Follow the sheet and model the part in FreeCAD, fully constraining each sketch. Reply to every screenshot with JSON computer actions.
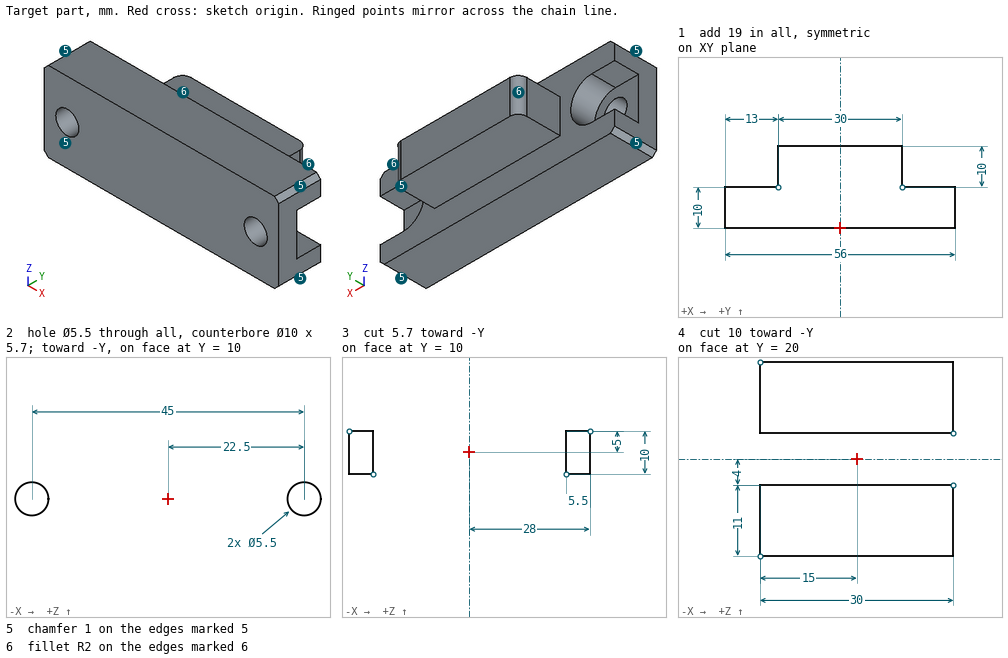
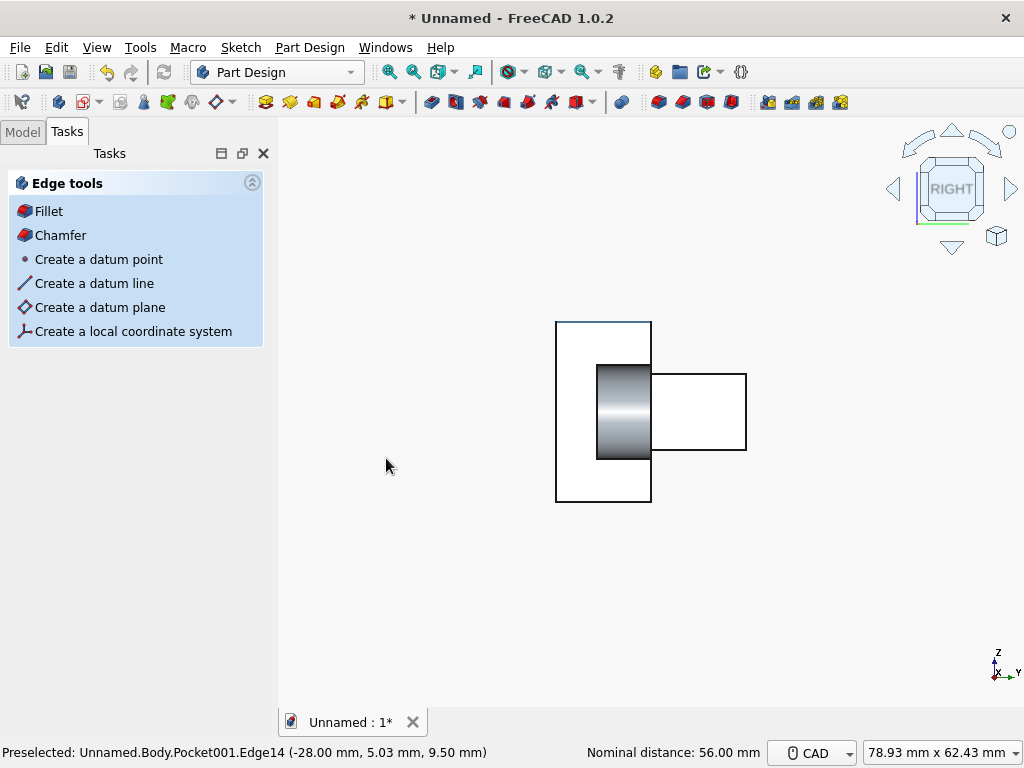
{"action": "left_click", "coordinate": [390, 72]}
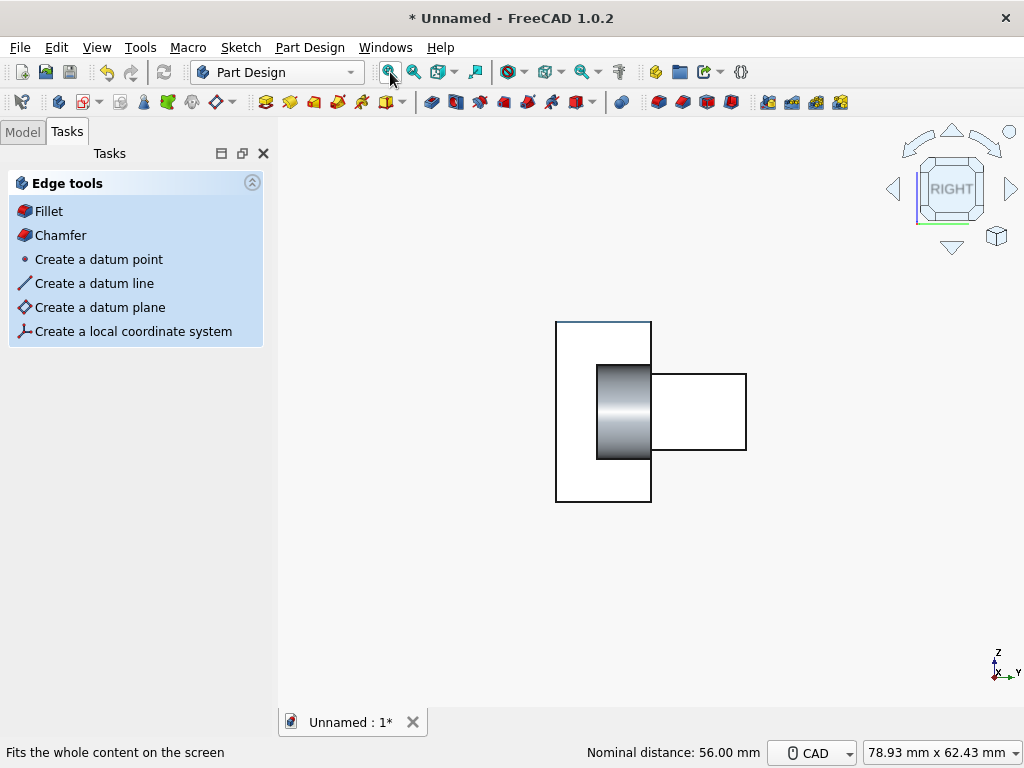
{"action": "left_click", "coordinate": [604, 501], "text": "ctrl"}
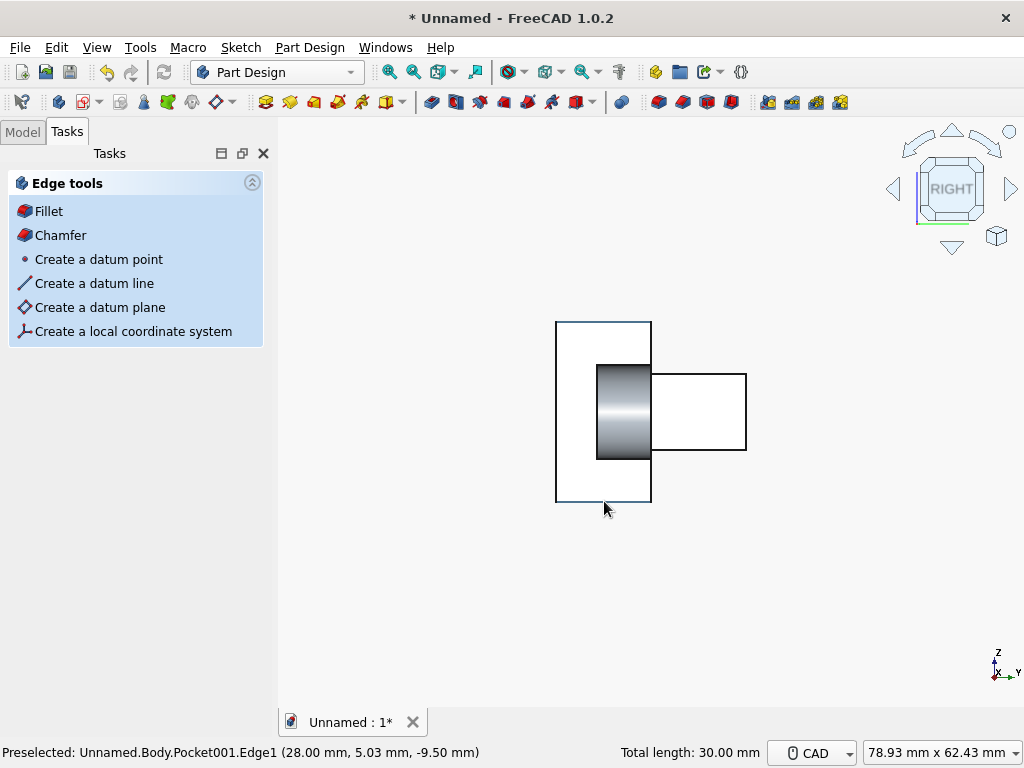
{"action": "key", "text": "5"}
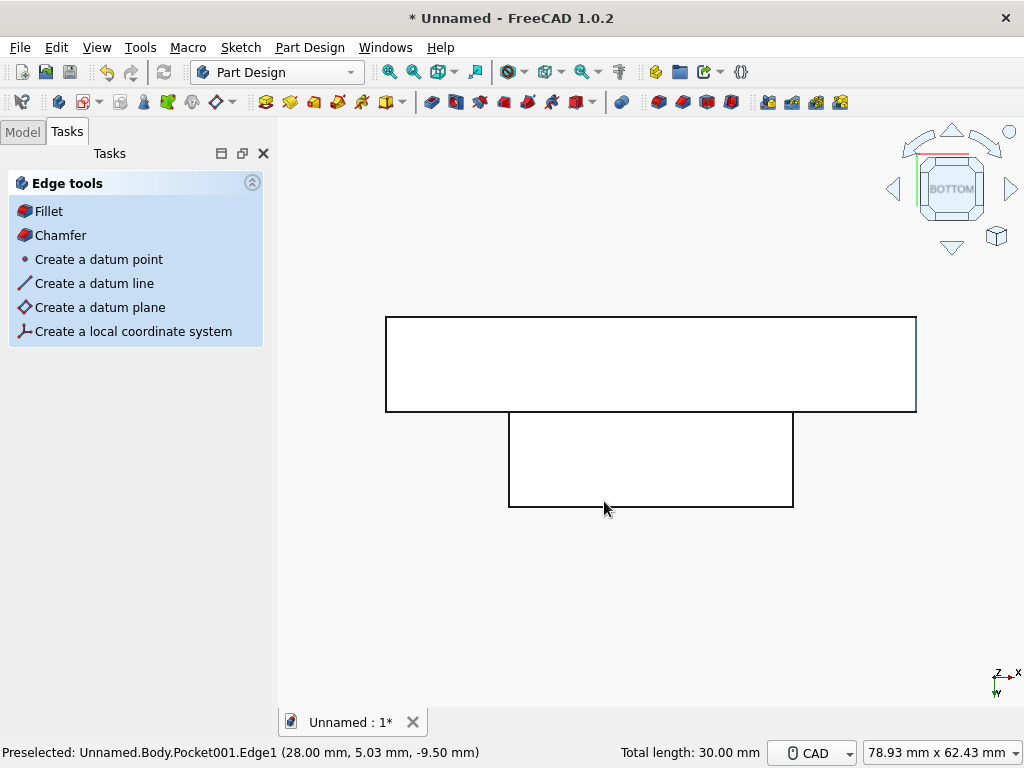
{"action": "left_click", "coordinate": [386, 364], "text": "ctrl"}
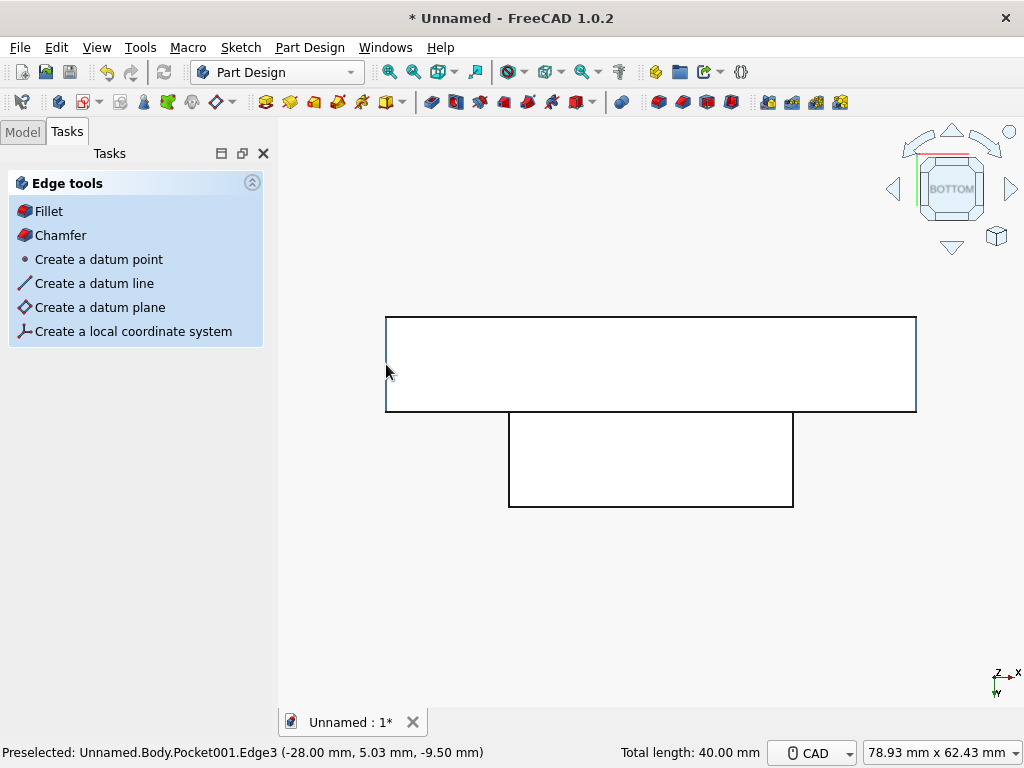
{"action": "left_click", "coordinate": [684, 102]}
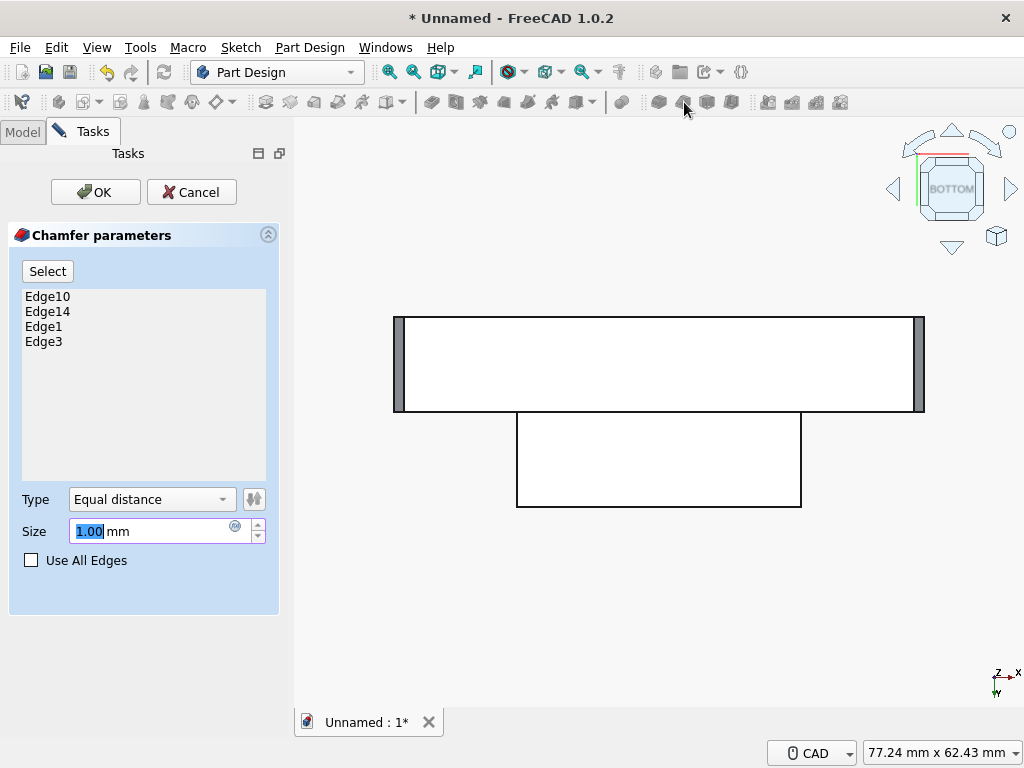
{"action": "type", "text": "1"}
{"action": "key", "text": "Tab"}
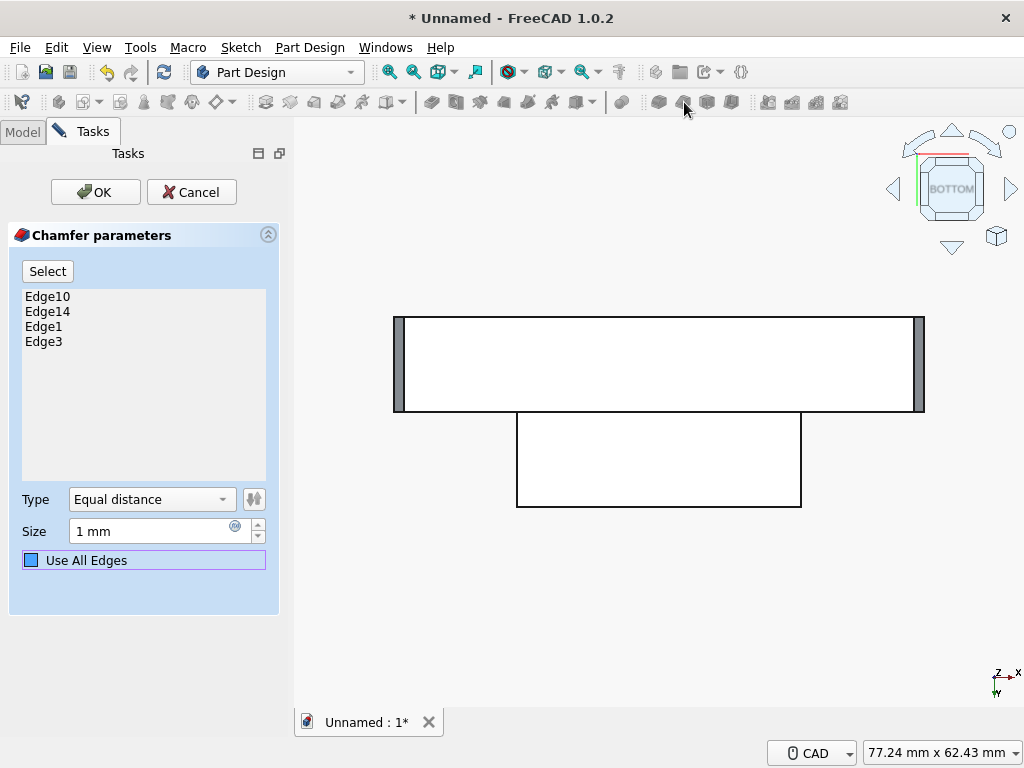
{"action": "left_click", "coordinate": [96, 192]}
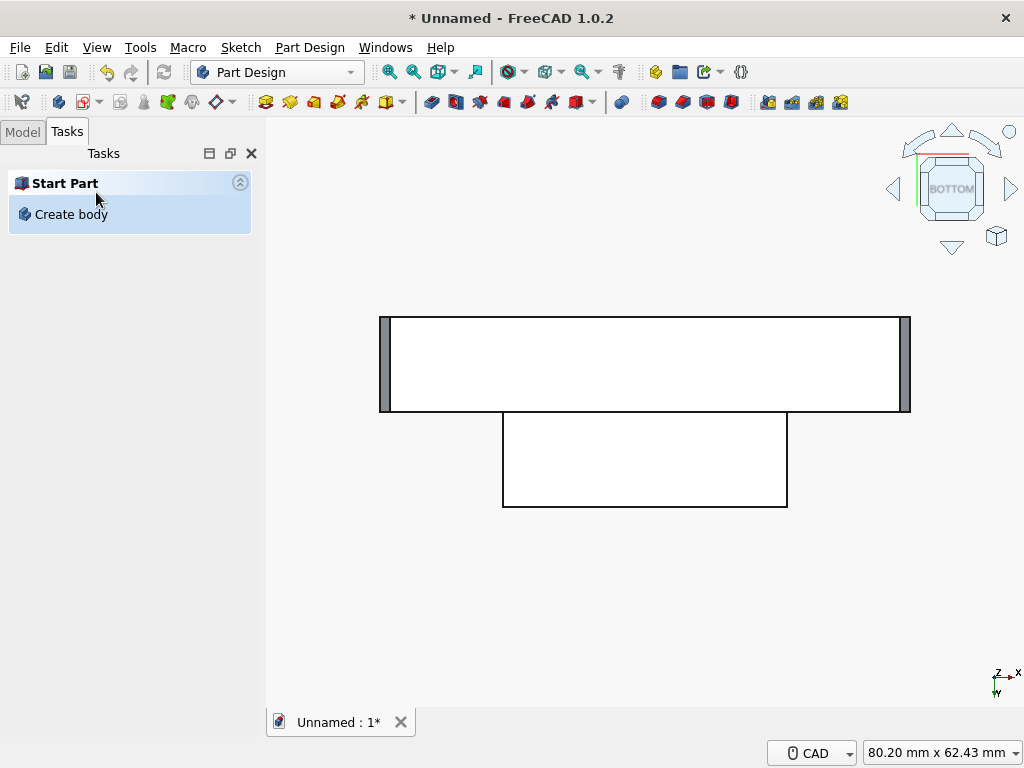
{"action": "key", "text": "0"}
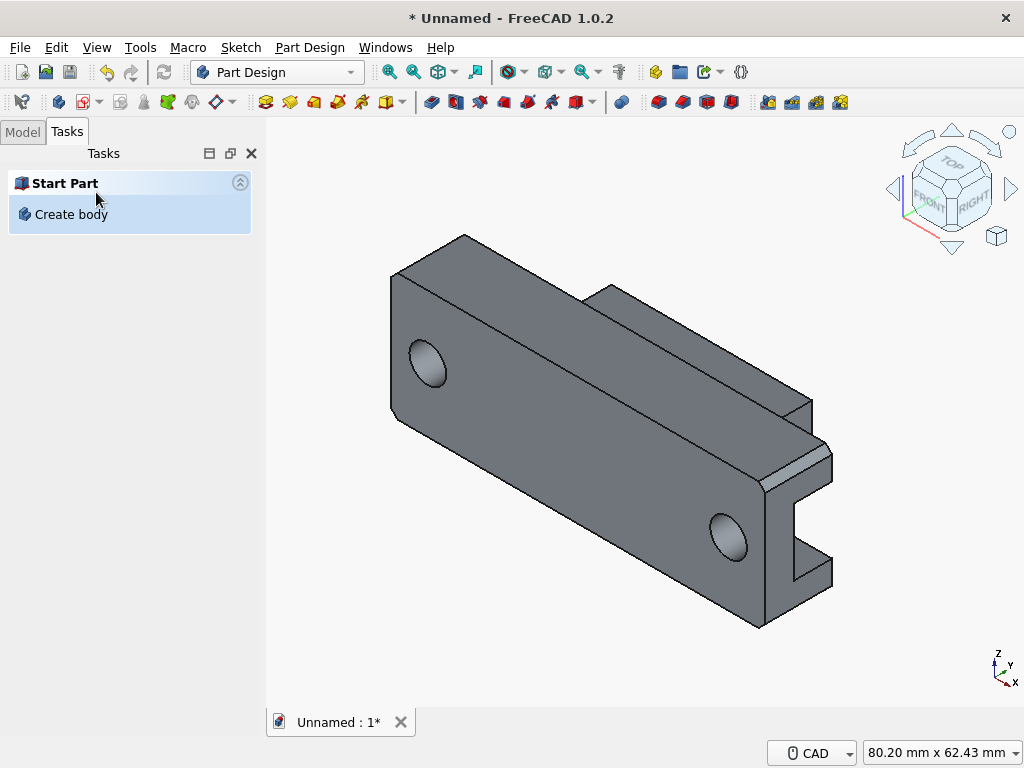
{"action": "key", "text": "2"}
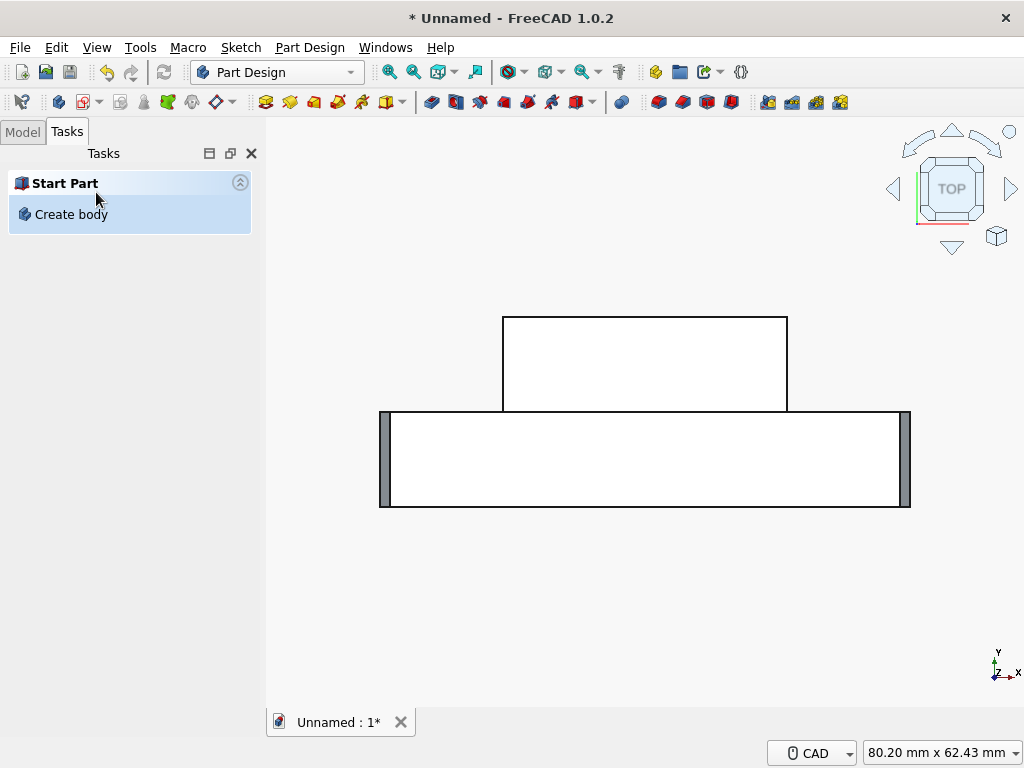
{"action": "key", "text": "1"}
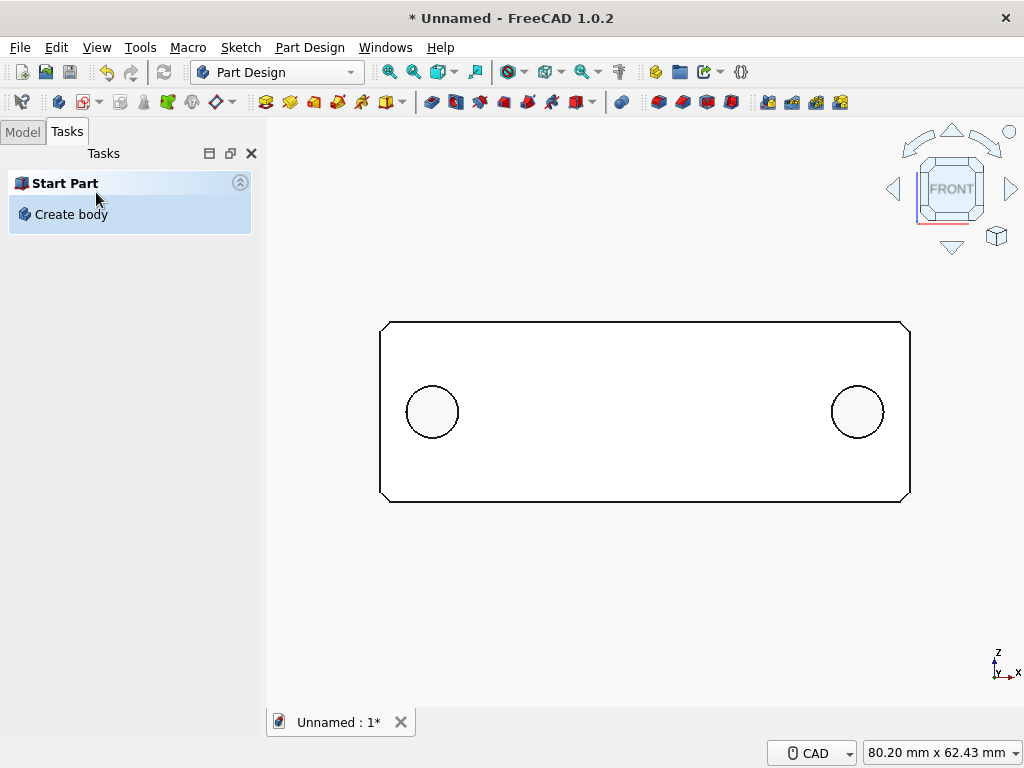
{"action": "key", "text": "3"}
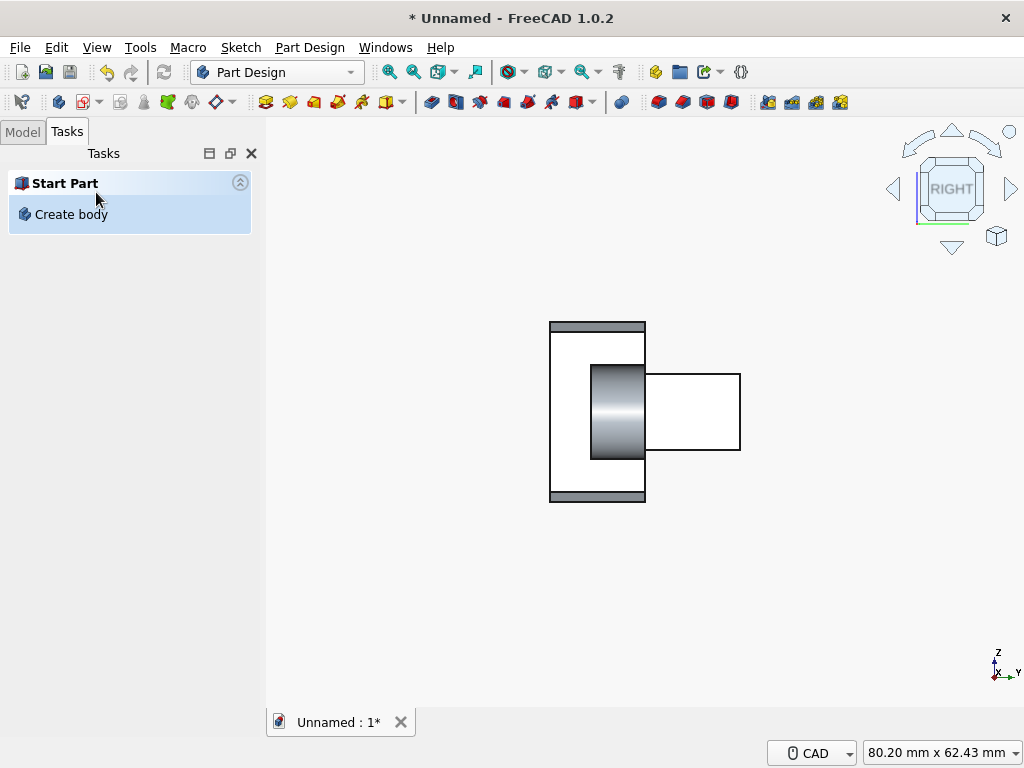
{"action": "key", "text": "v f"}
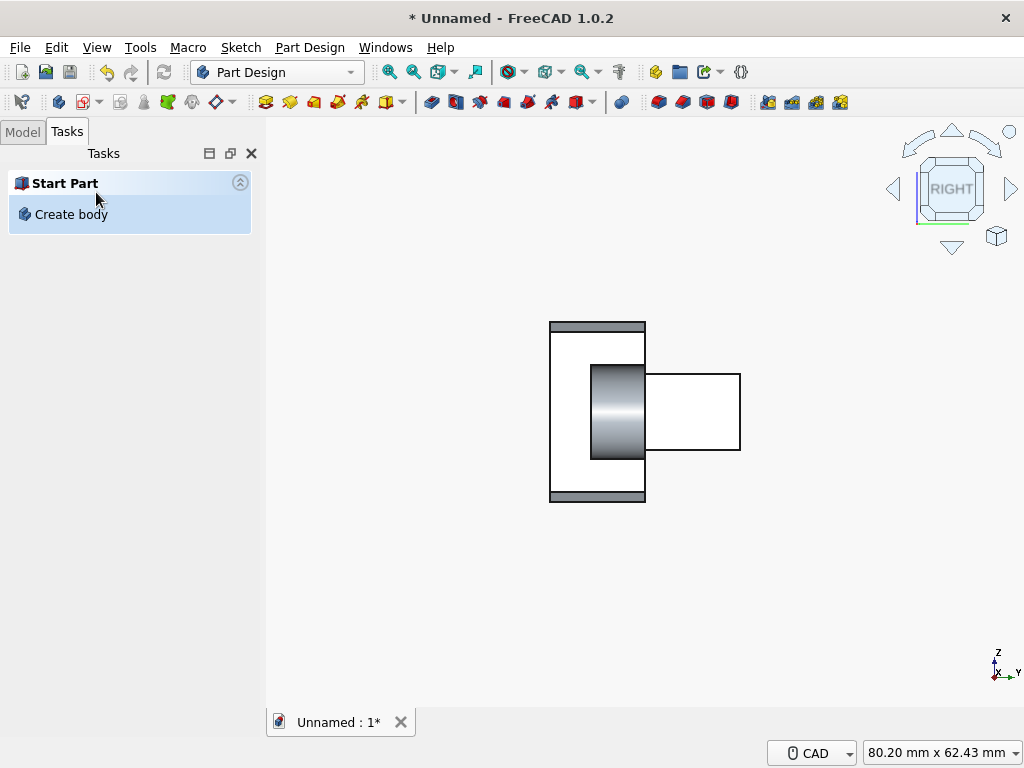
{"action": "left_click", "coordinate": [740, 411]}